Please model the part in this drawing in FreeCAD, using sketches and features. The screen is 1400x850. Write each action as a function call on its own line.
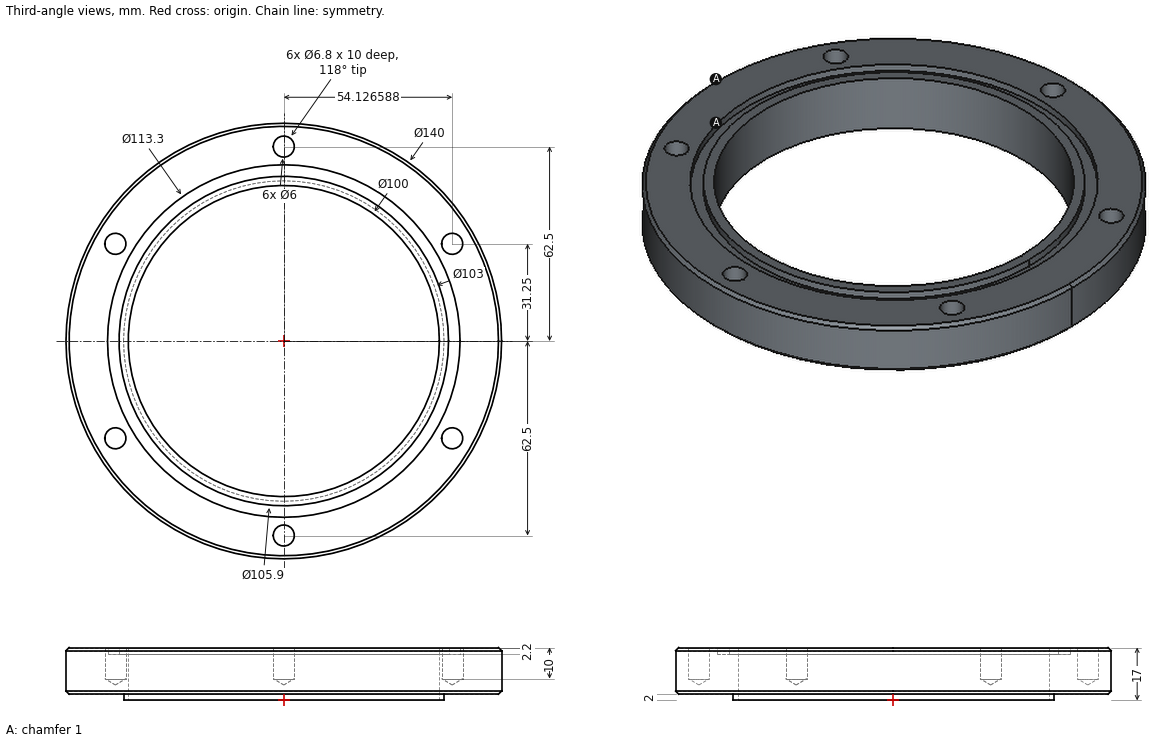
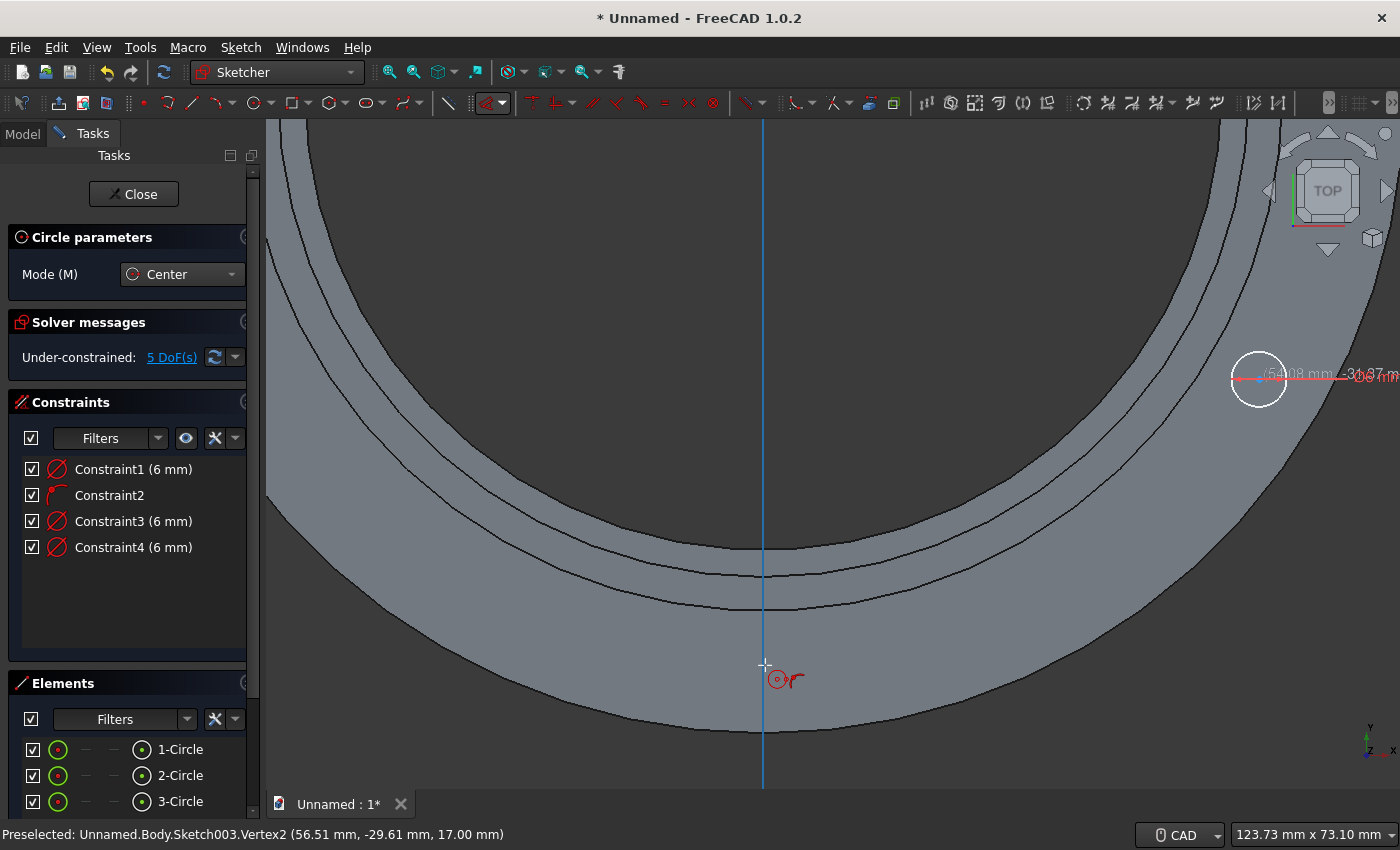
click(763, 665)
move(783, 645)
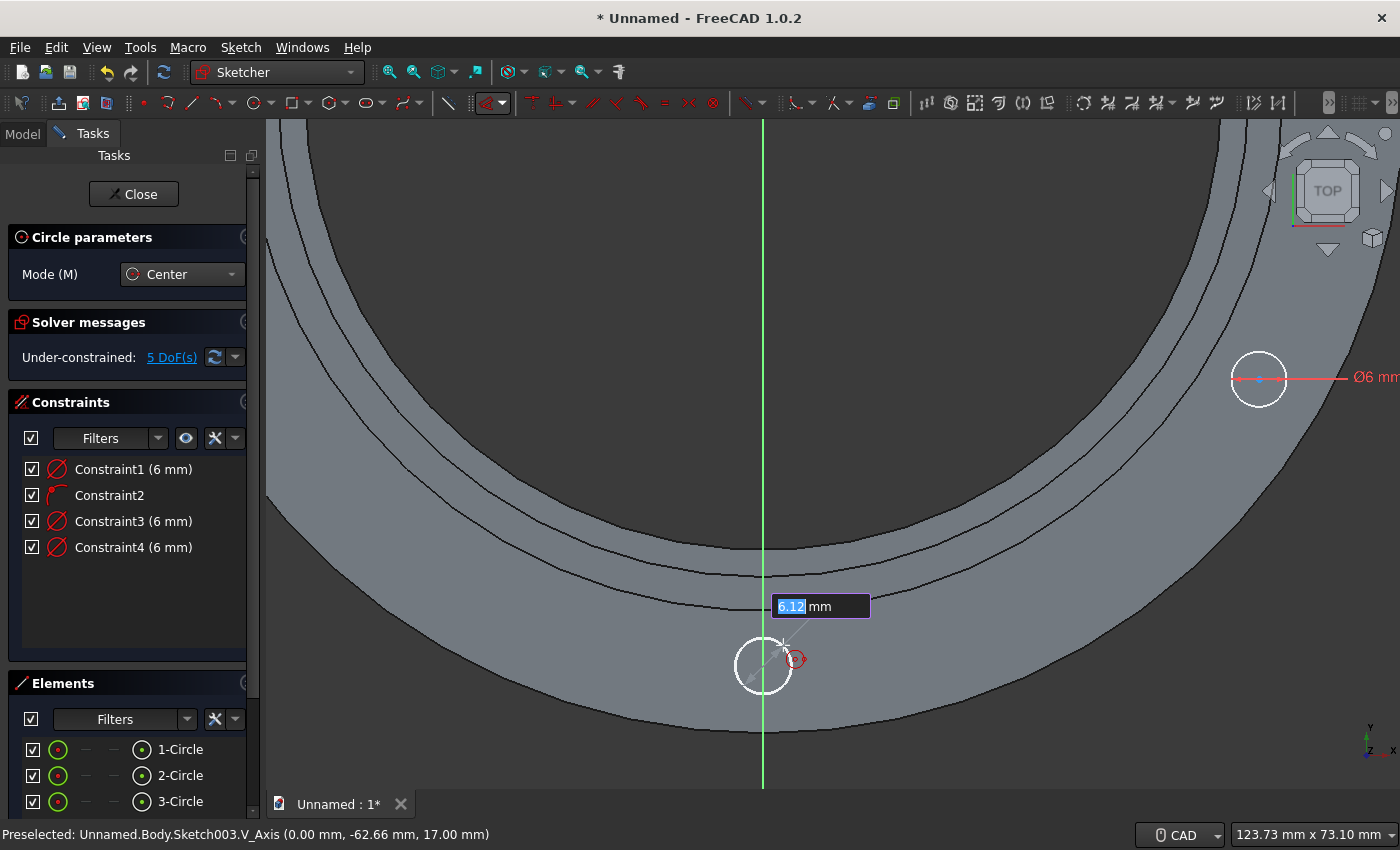
text(6)
key(Return)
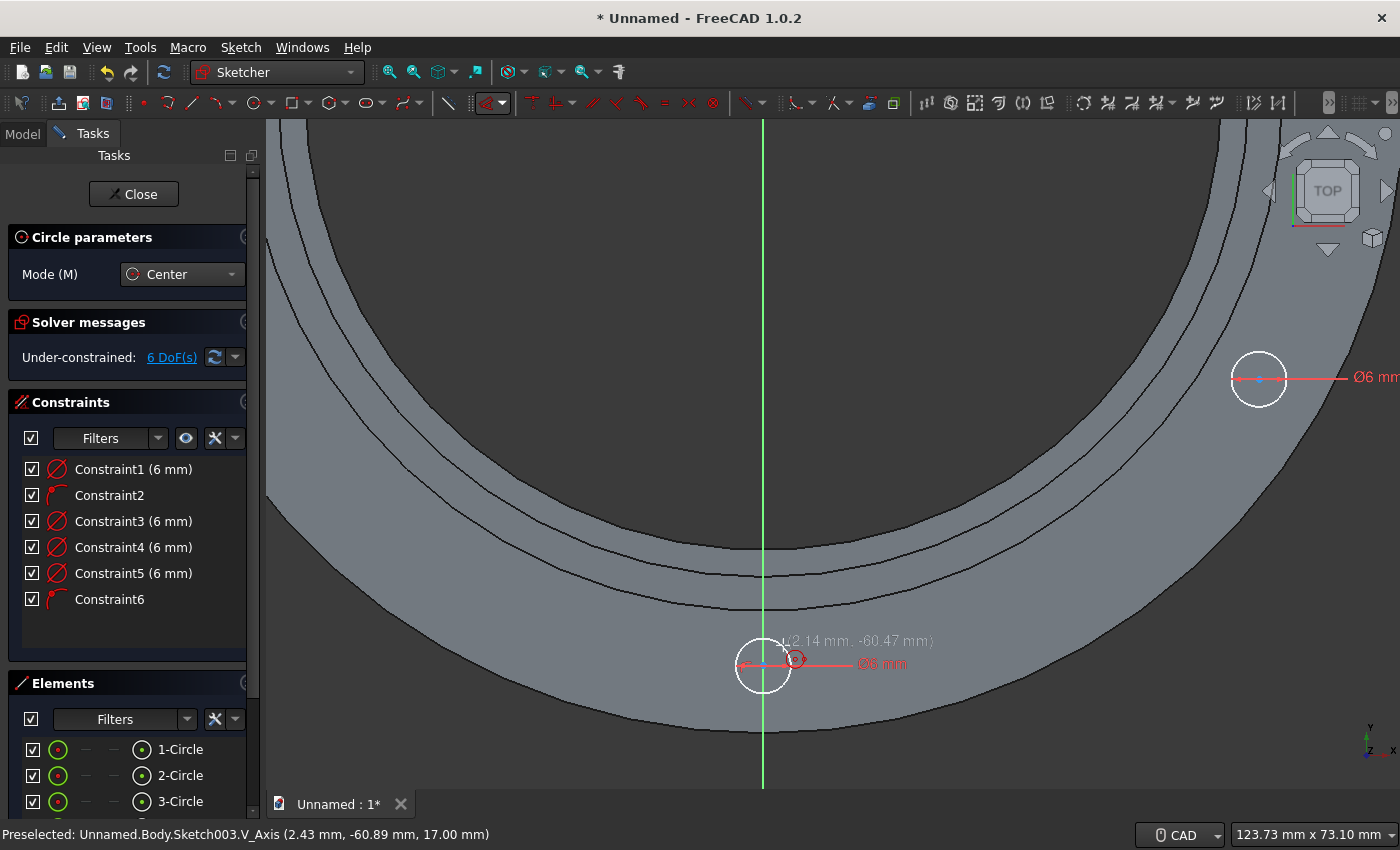
scroll(765, 665, down, 5)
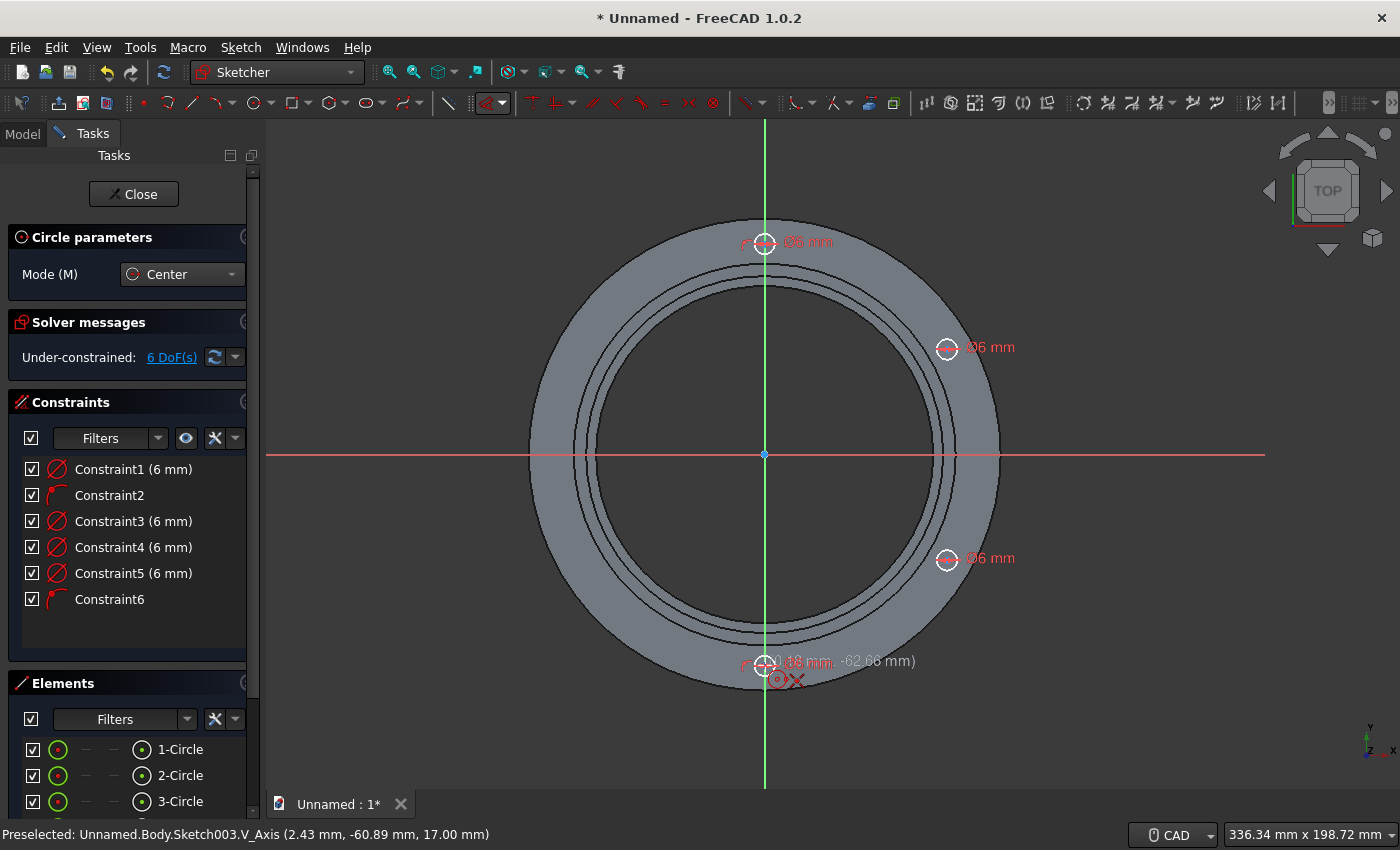
scroll(582, 560, up, 5)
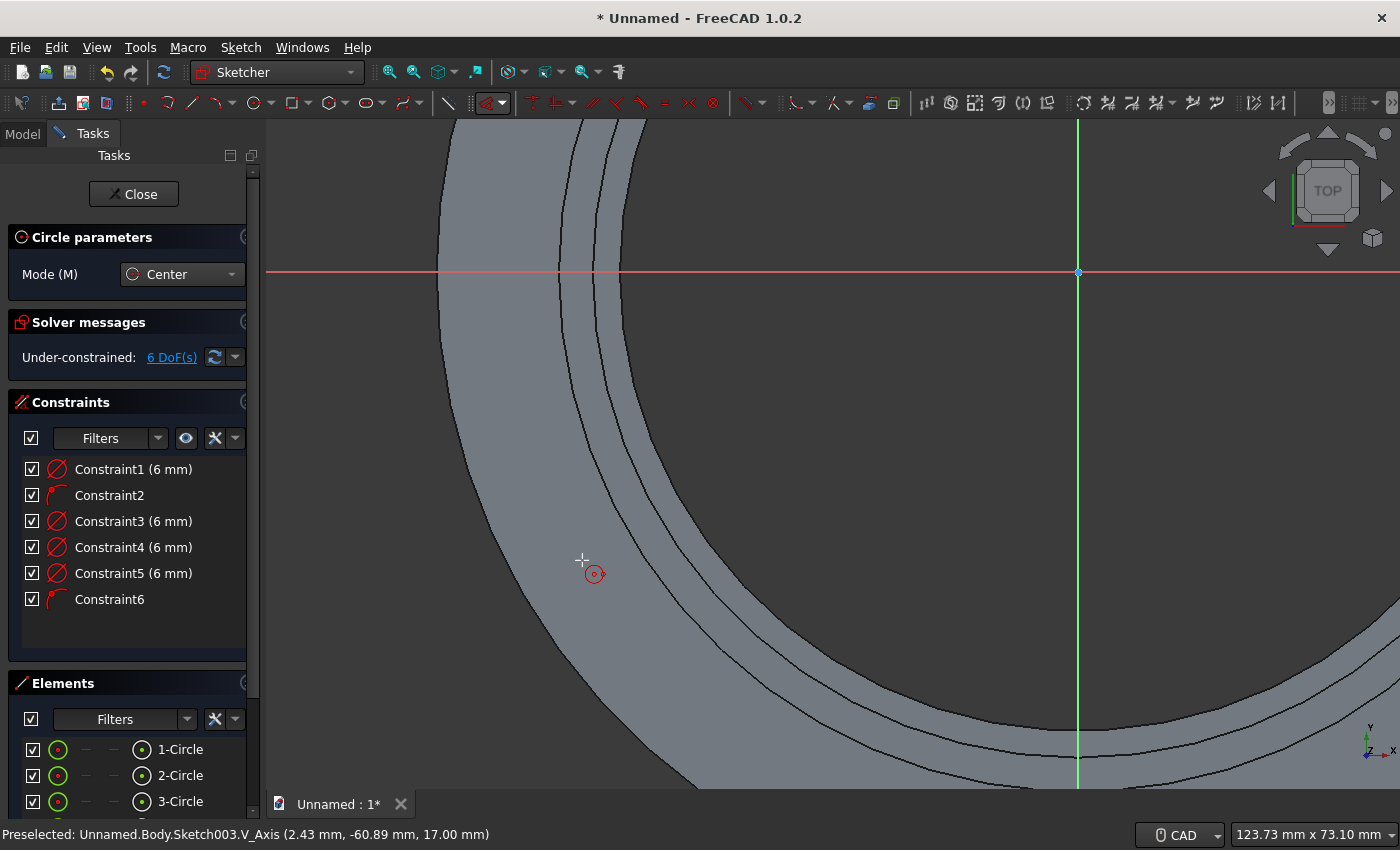
click(582, 559)
move(601, 539)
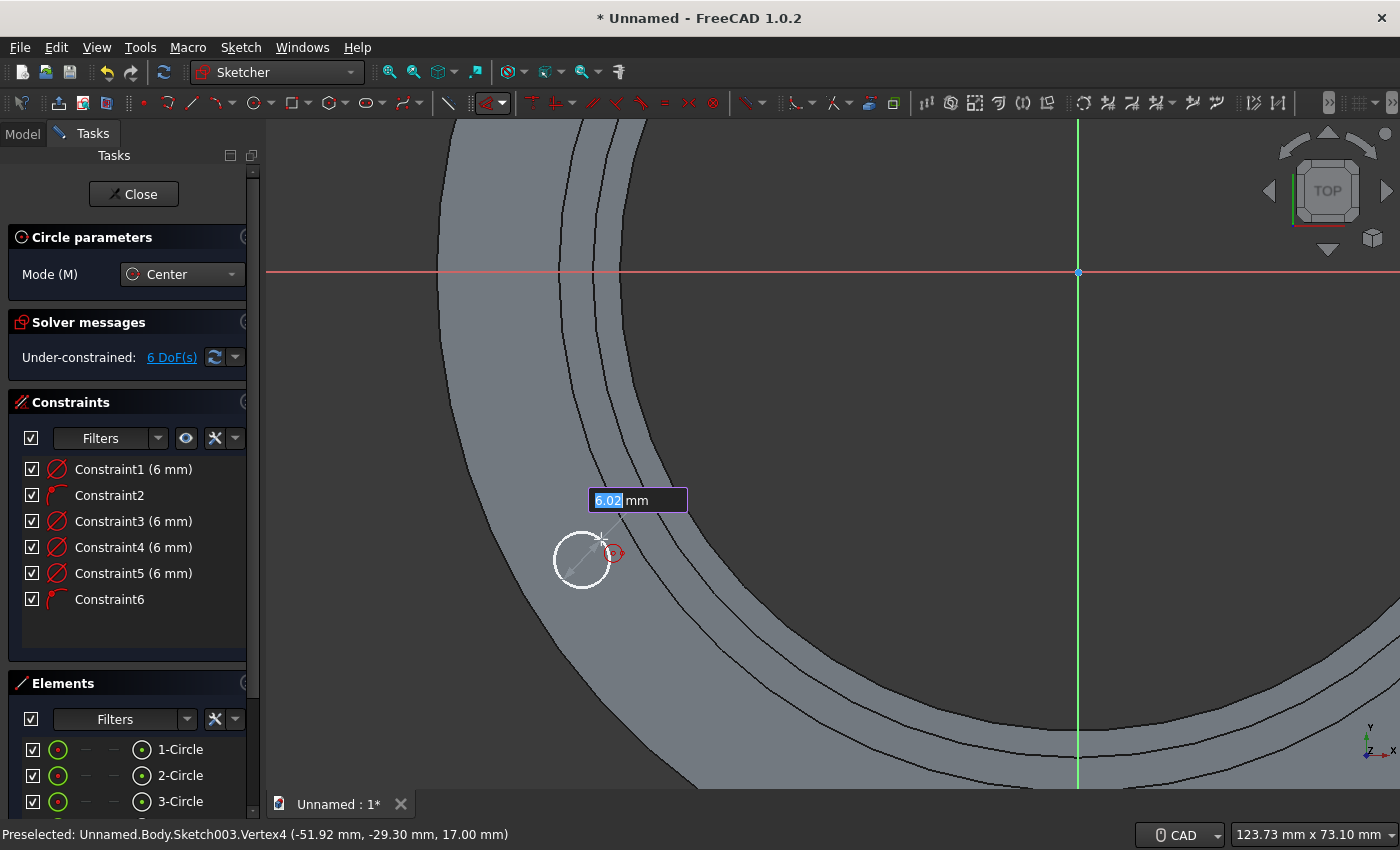
text(6)
key(Return)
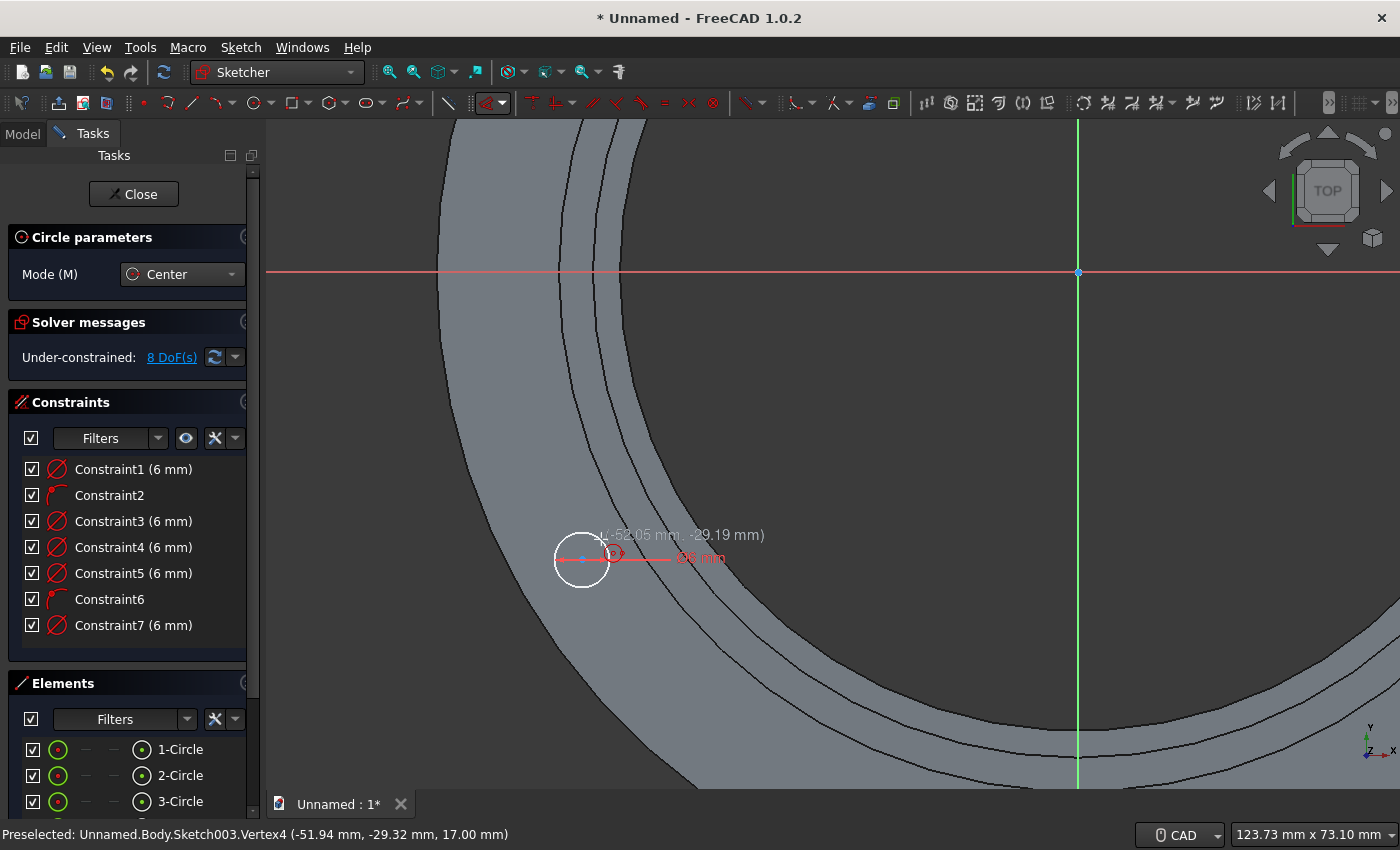
scroll(582, 560, down, 5)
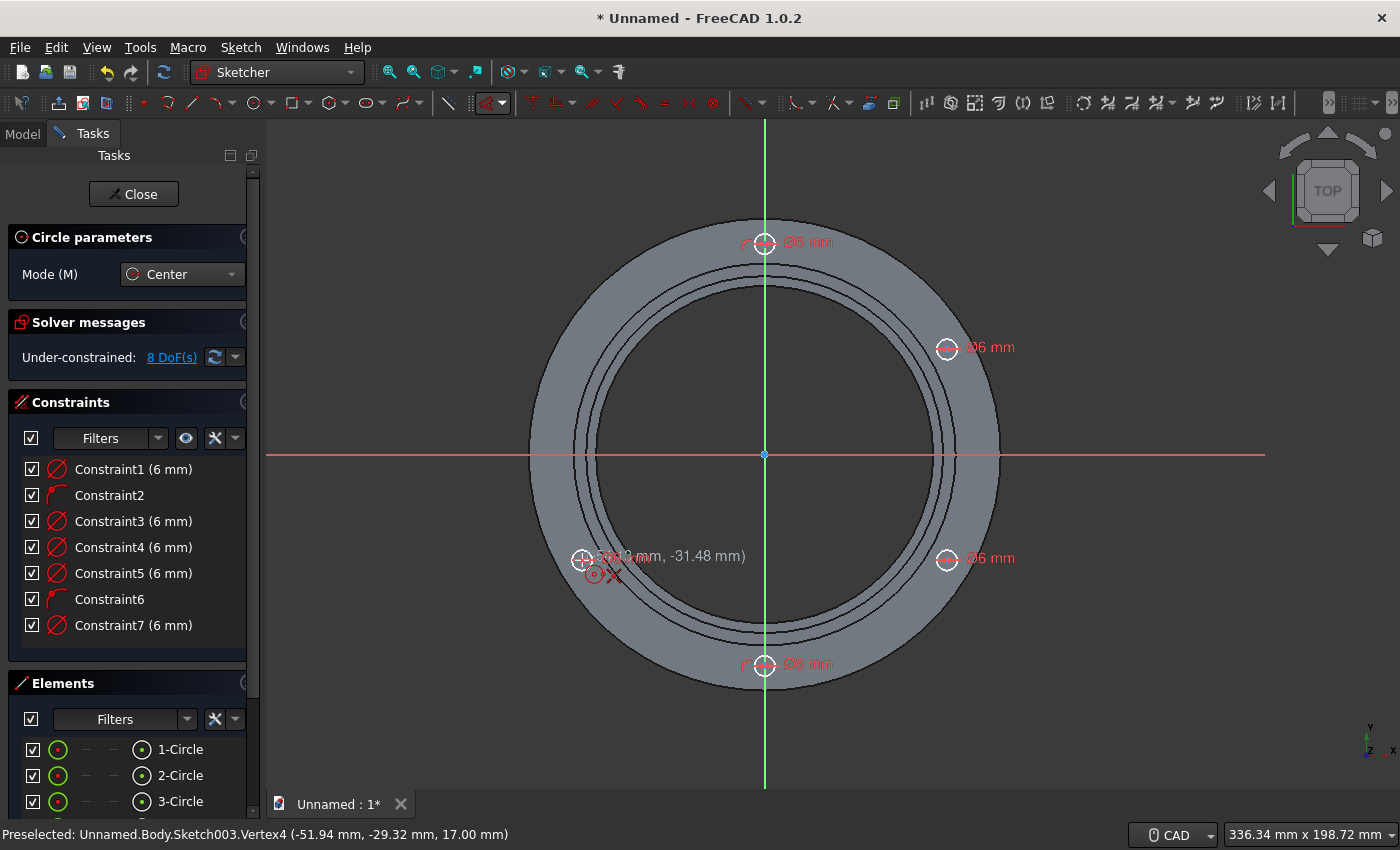
scroll(582, 349, up, 5)